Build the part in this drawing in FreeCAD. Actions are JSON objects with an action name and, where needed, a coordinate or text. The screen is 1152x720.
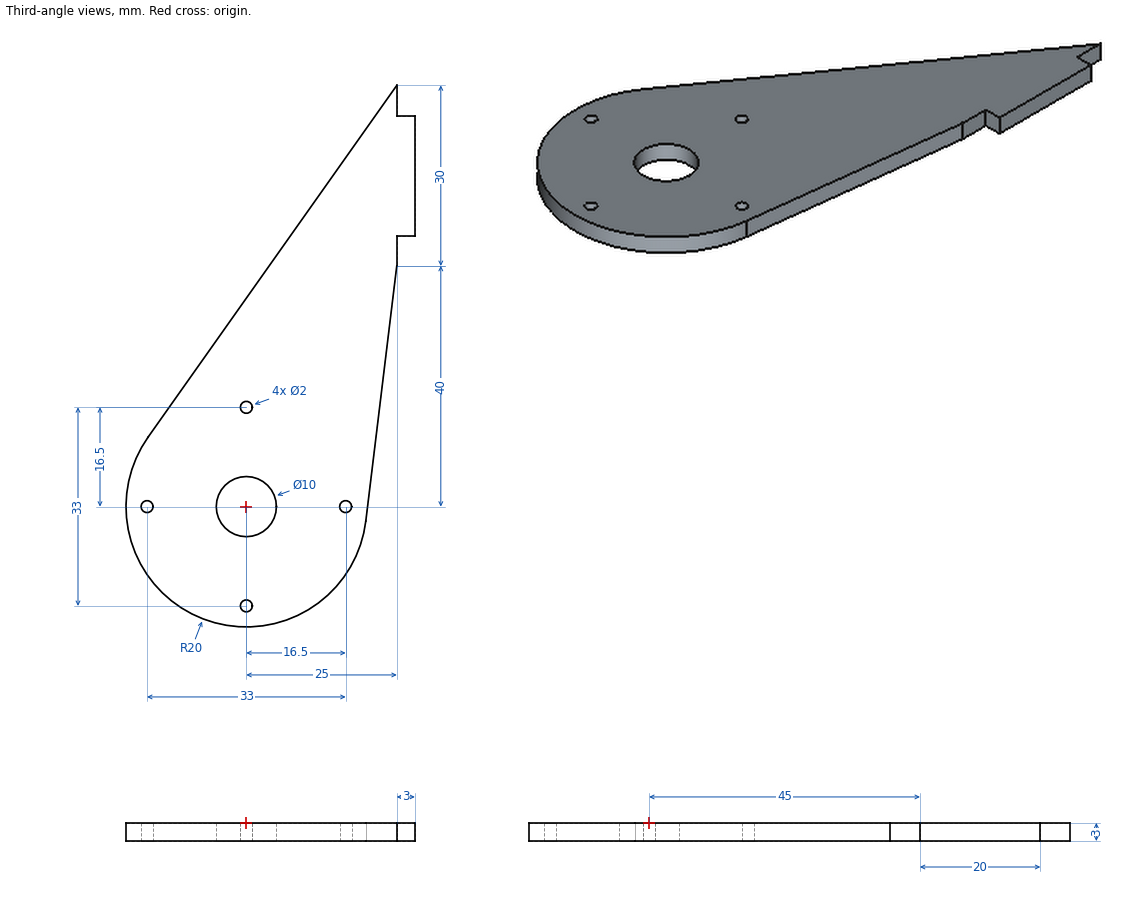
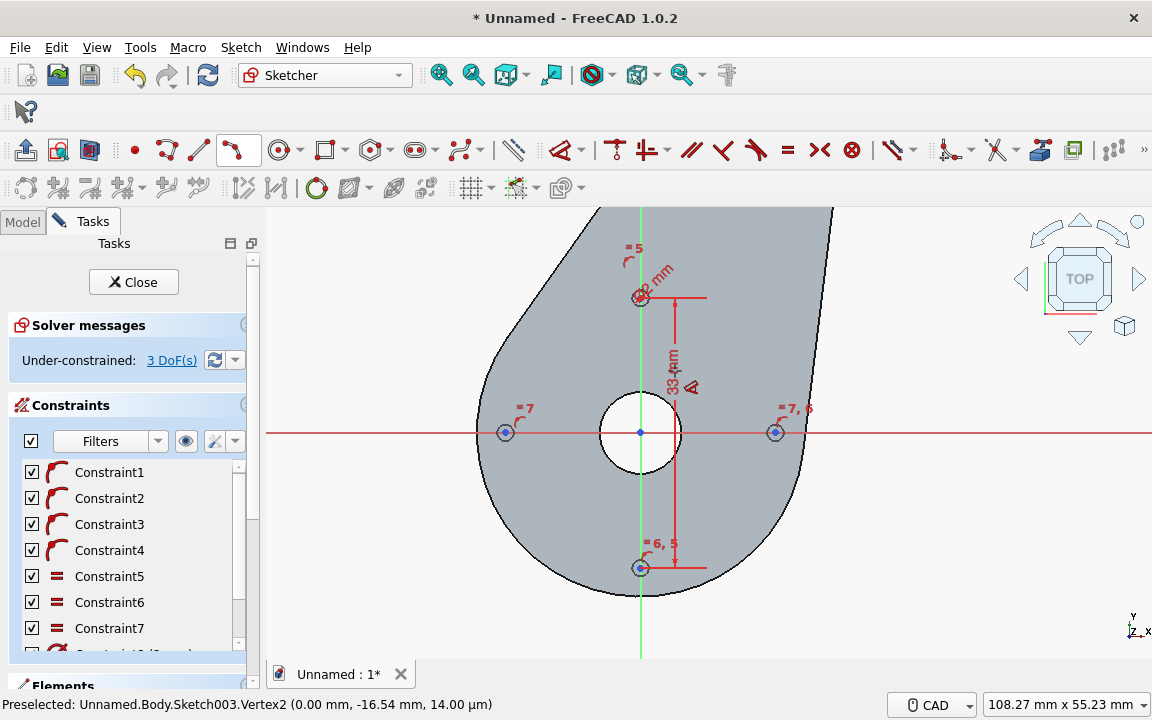
{"action": "left_click", "coordinate": [775, 433]}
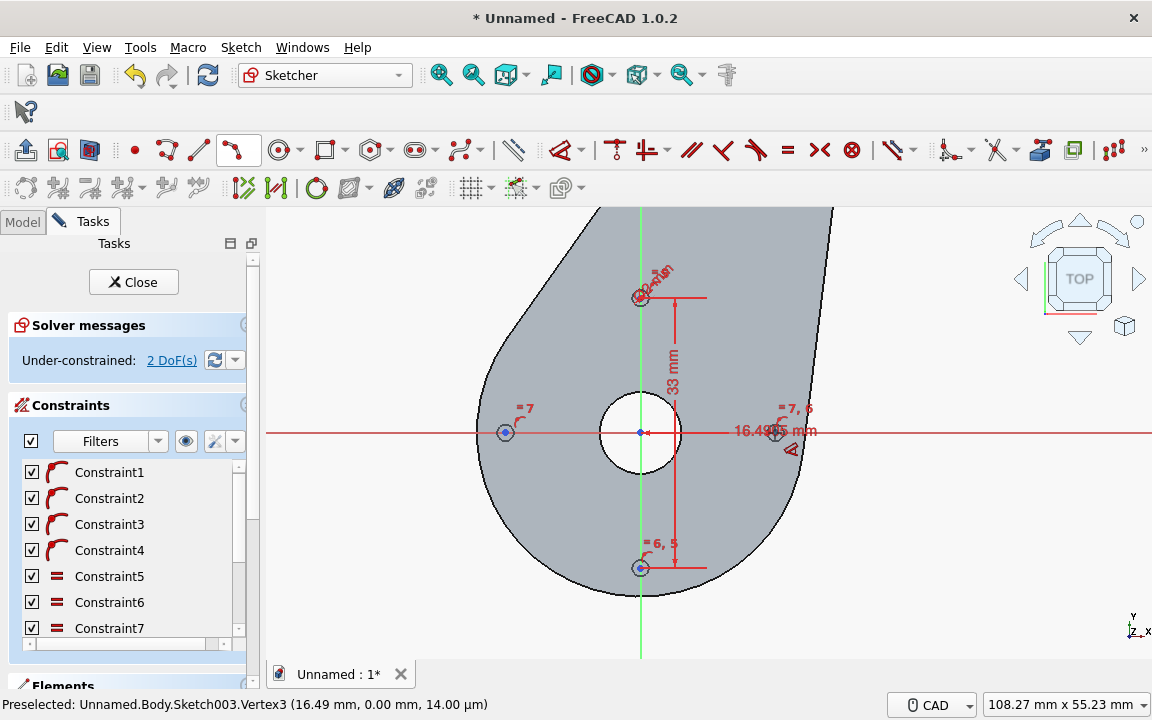
{"action": "left_click", "coordinate": [505, 433]}
{"action": "left_click", "coordinate": [578, 467]}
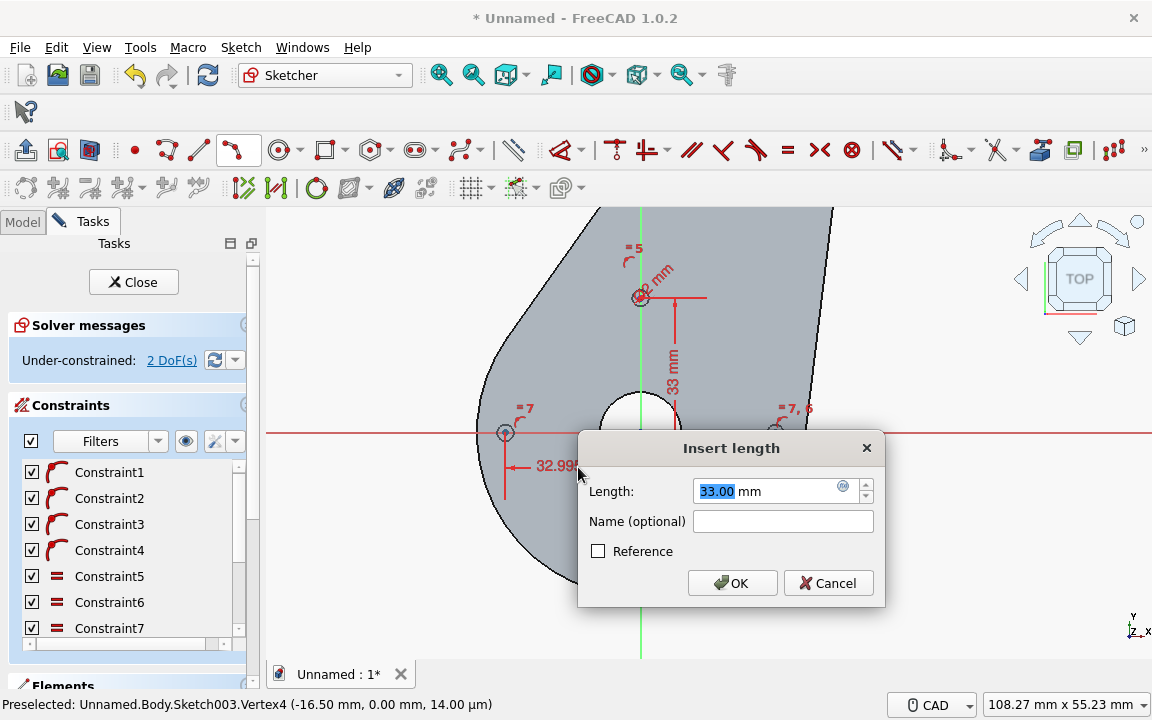
{"action": "type", "text": "33"}
{"action": "key", "text": "Return"}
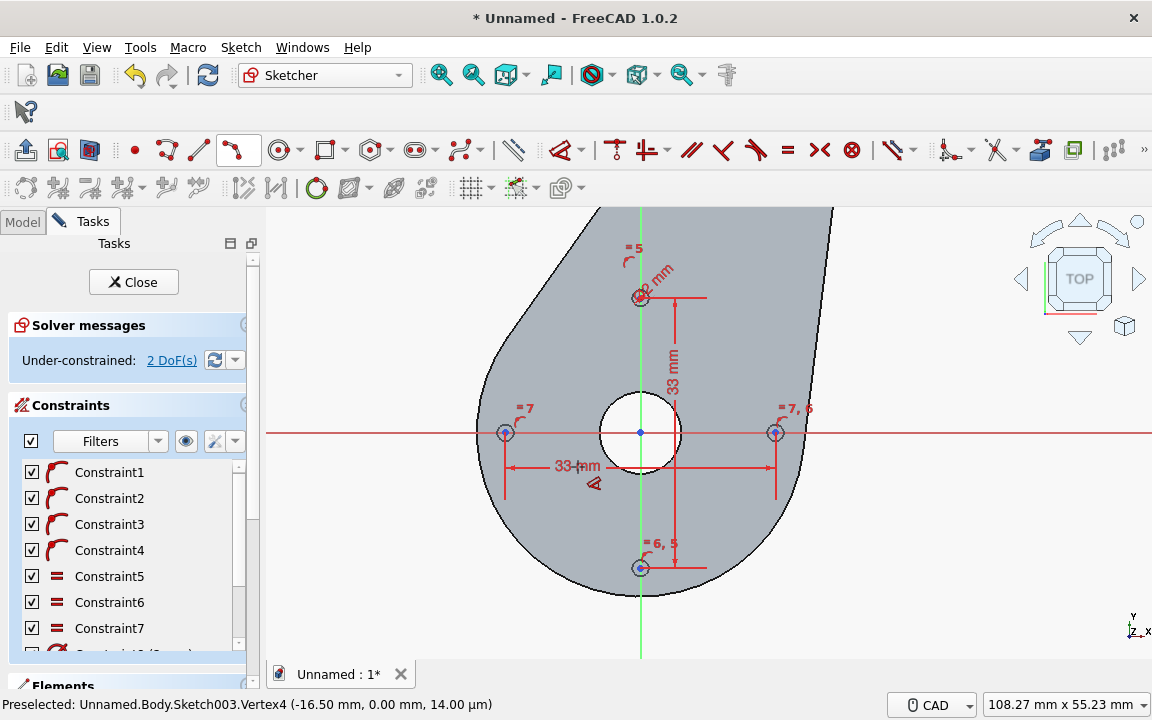
{"action": "left_click", "coordinate": [641, 298]}
{"action": "left_click", "coordinate": [675, 335]}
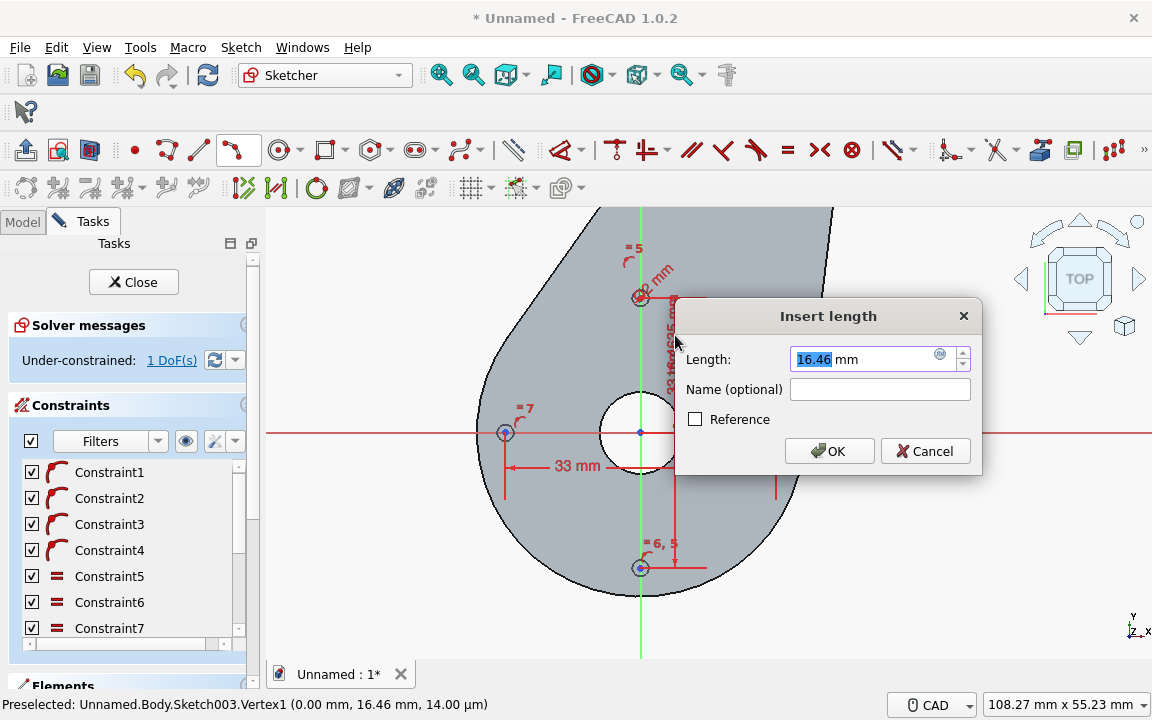
{"action": "type", "text": "16.5"}
{"action": "key", "text": "Return"}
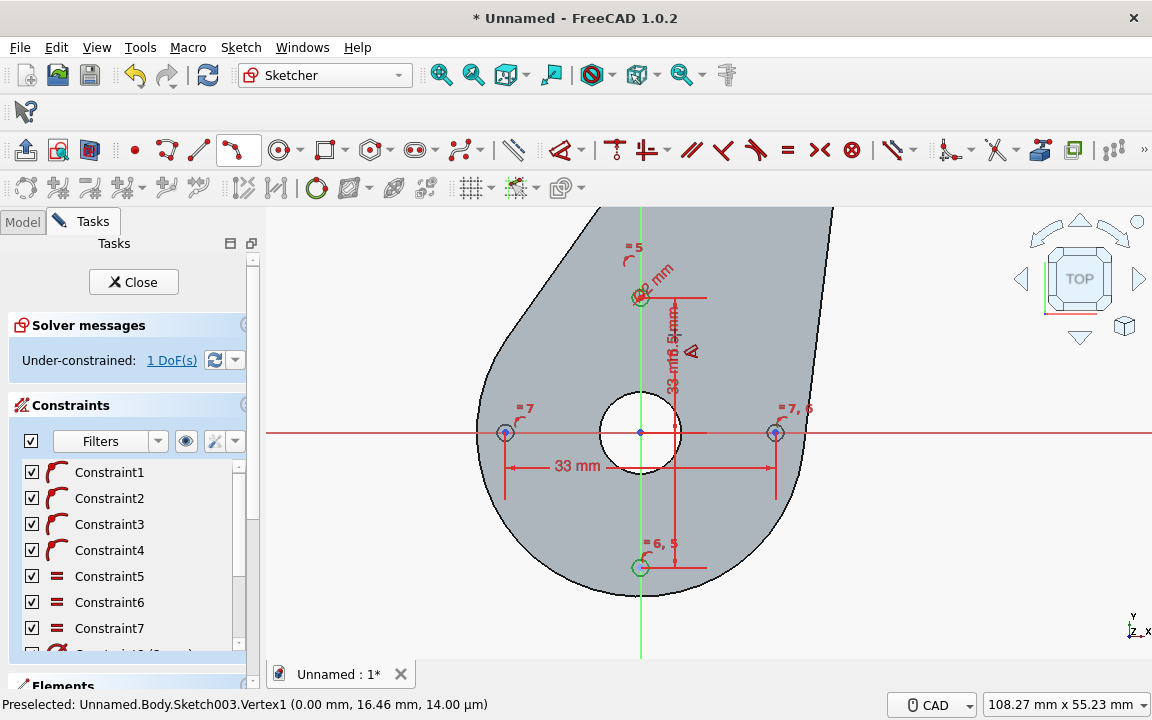
{"action": "left_click", "coordinate": [776, 433]}
{"action": "left_click", "coordinate": [708, 467]}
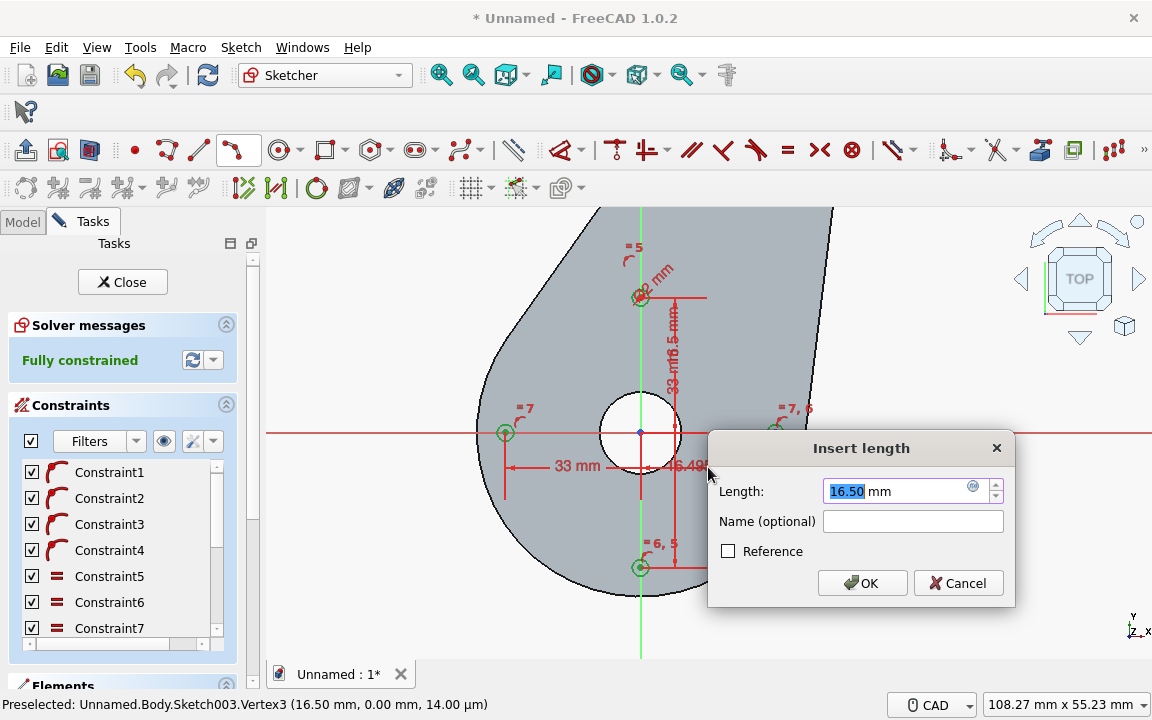
{"action": "type", "text": "16.5"}
{"action": "key", "text": "Return"}
{"action": "key", "text": "Escape"}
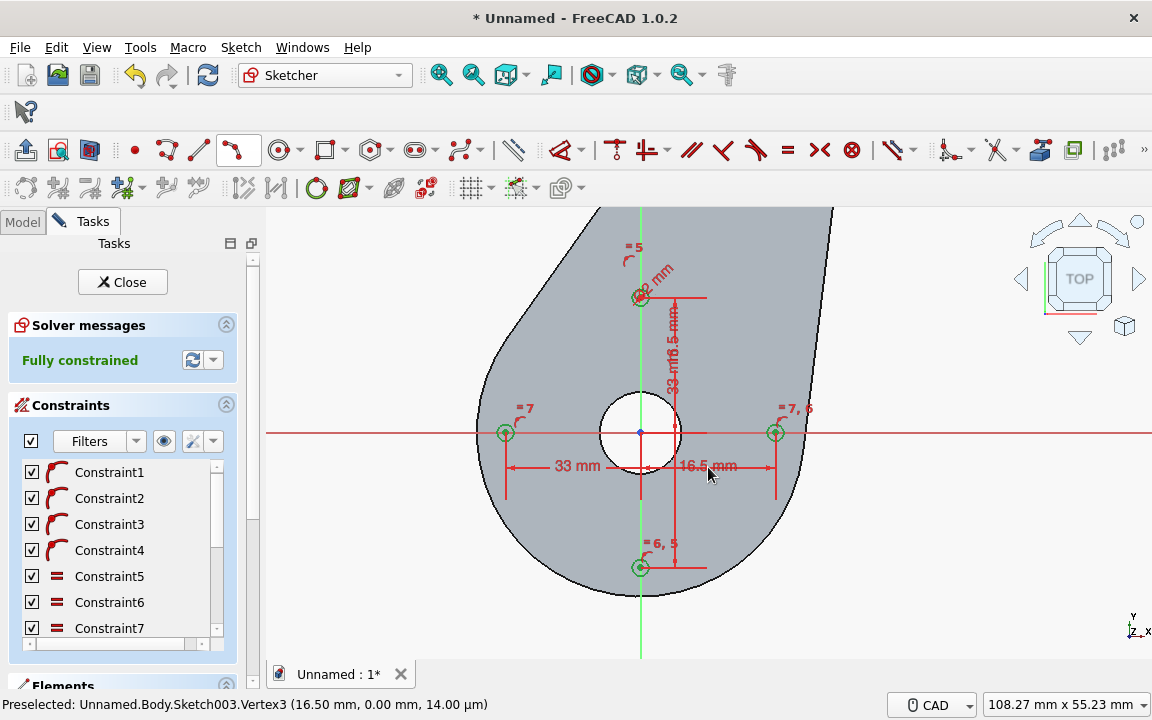
{"action": "left_click", "coordinate": [123, 282]}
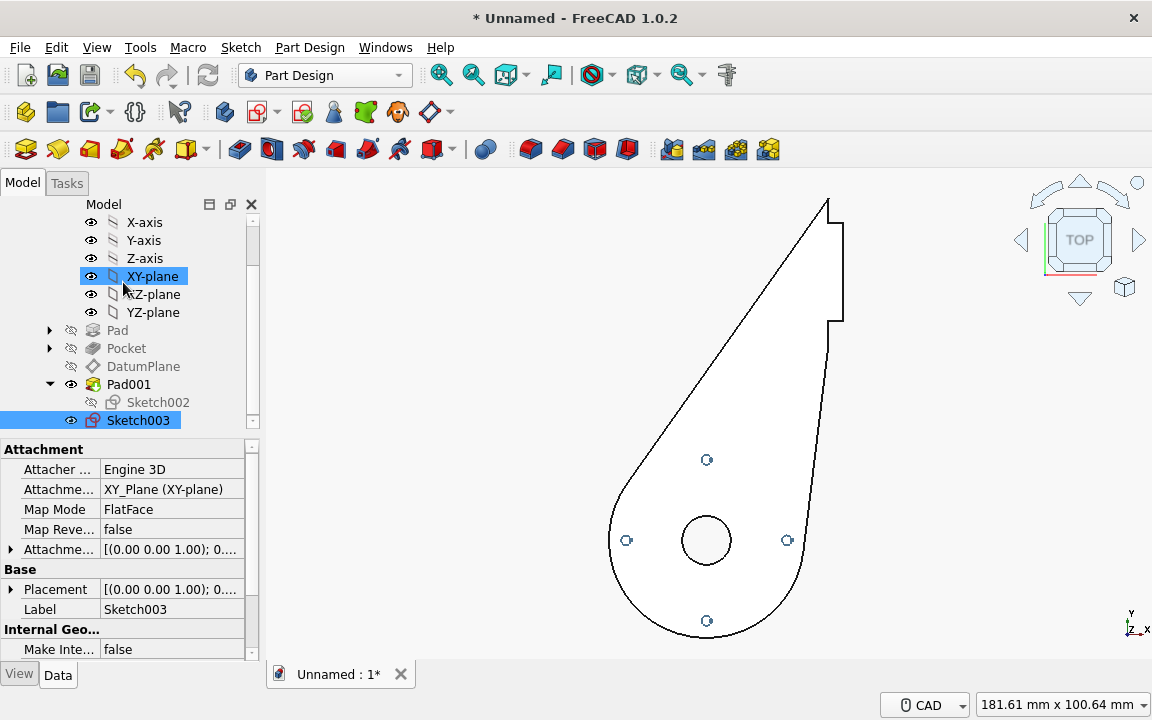
{"action": "left_click", "coordinate": [240, 150]}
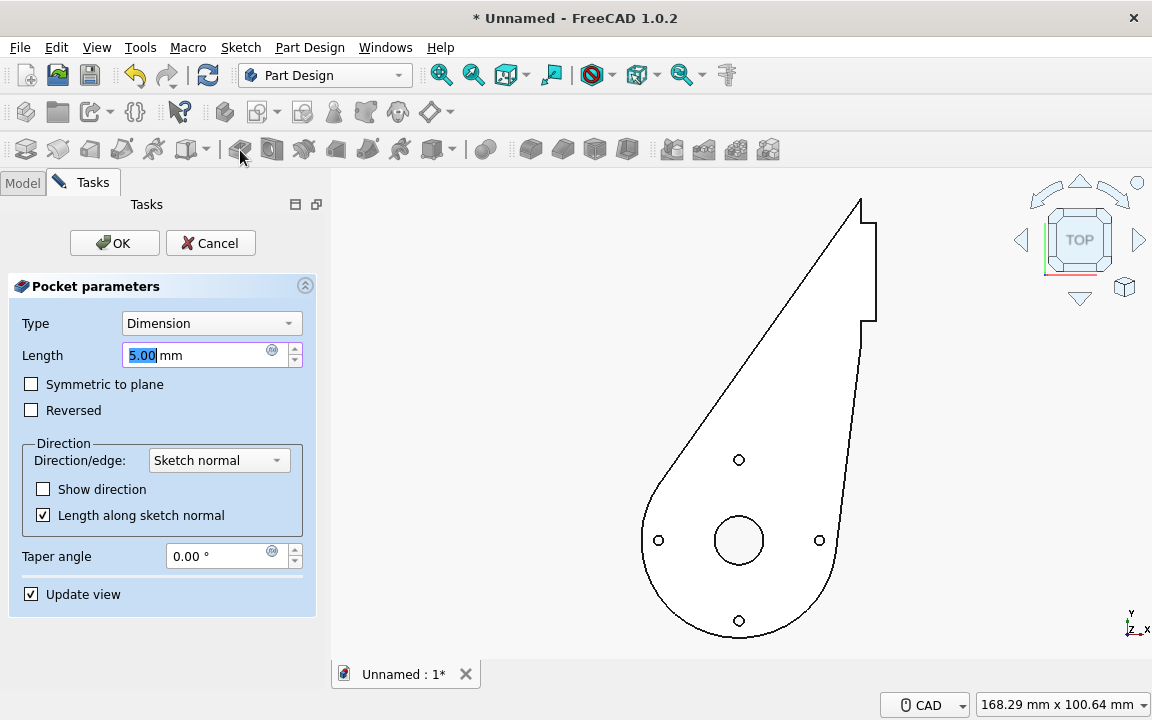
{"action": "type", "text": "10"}
{"action": "key", "text": "Tab"}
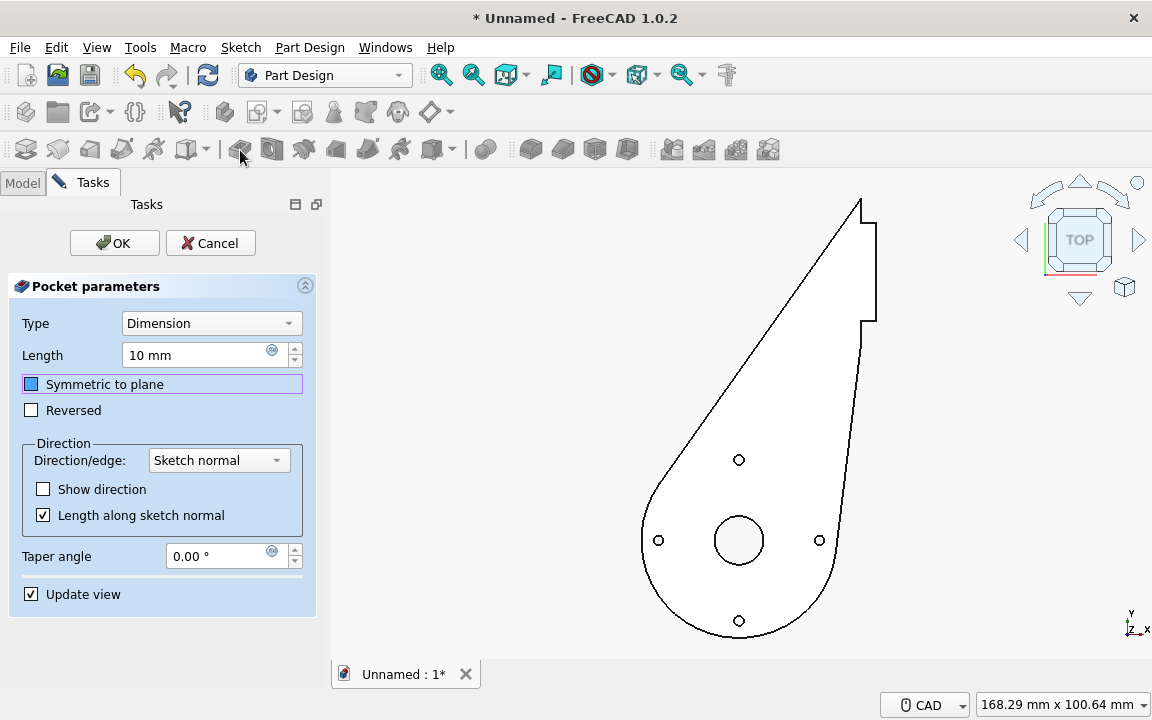
{"action": "left_click", "coordinate": [115, 243]}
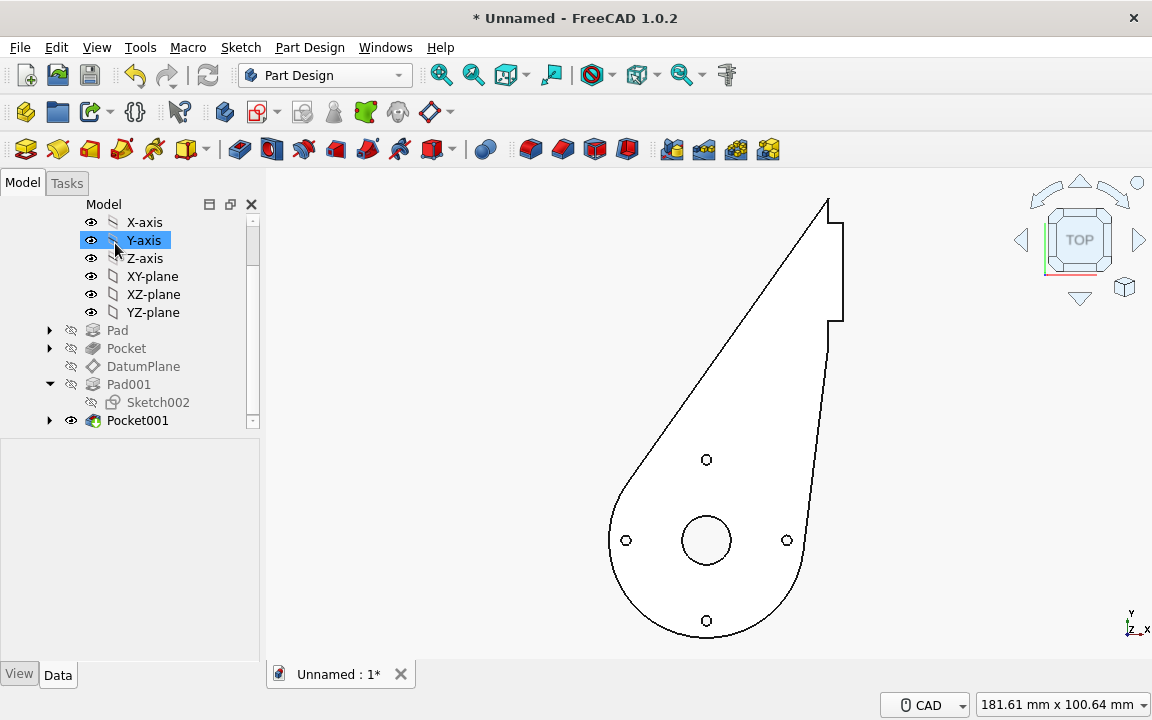
{"action": "key", "text": "0"}